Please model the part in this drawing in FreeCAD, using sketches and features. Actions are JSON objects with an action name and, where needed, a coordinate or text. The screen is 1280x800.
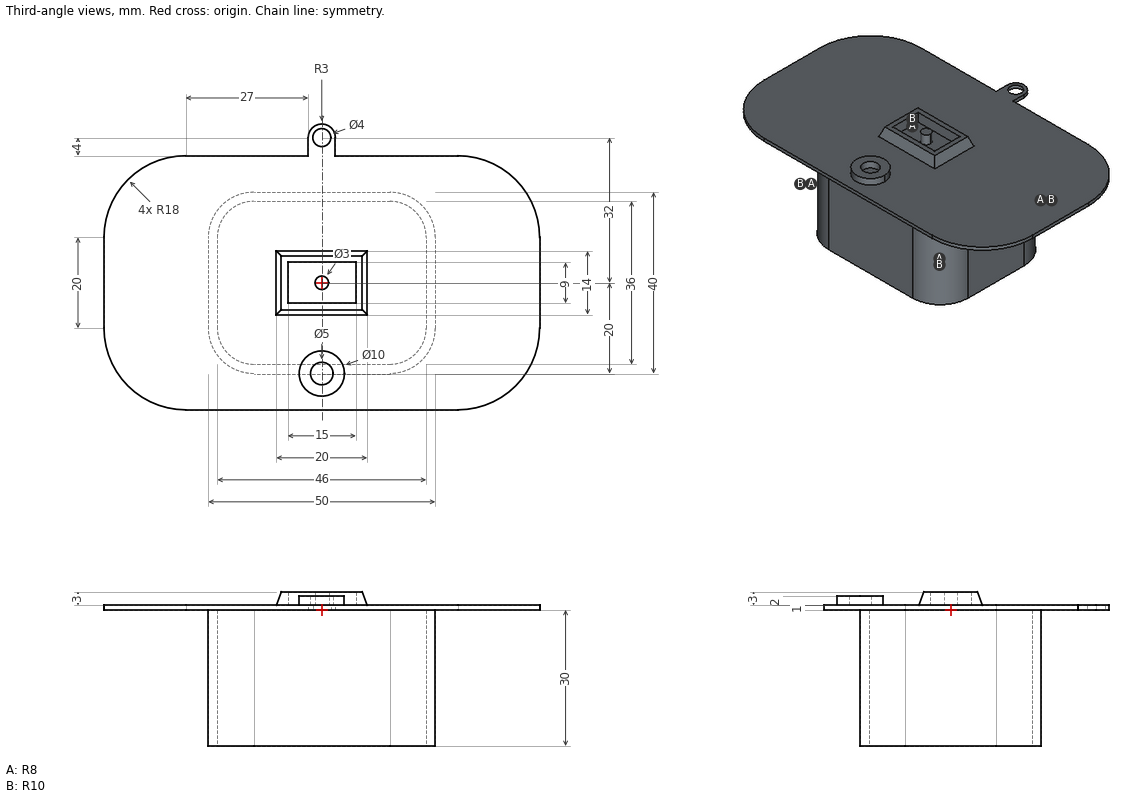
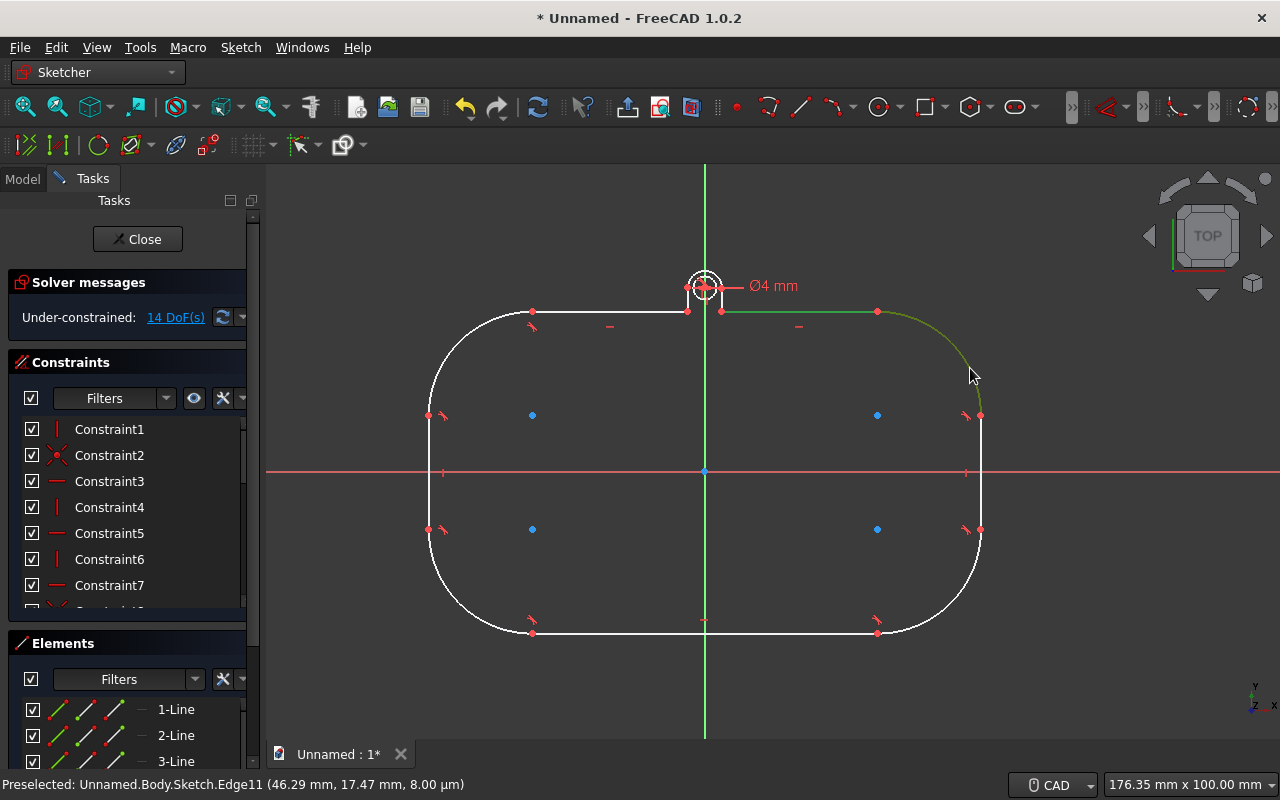
{"action": "key", "text": "t"}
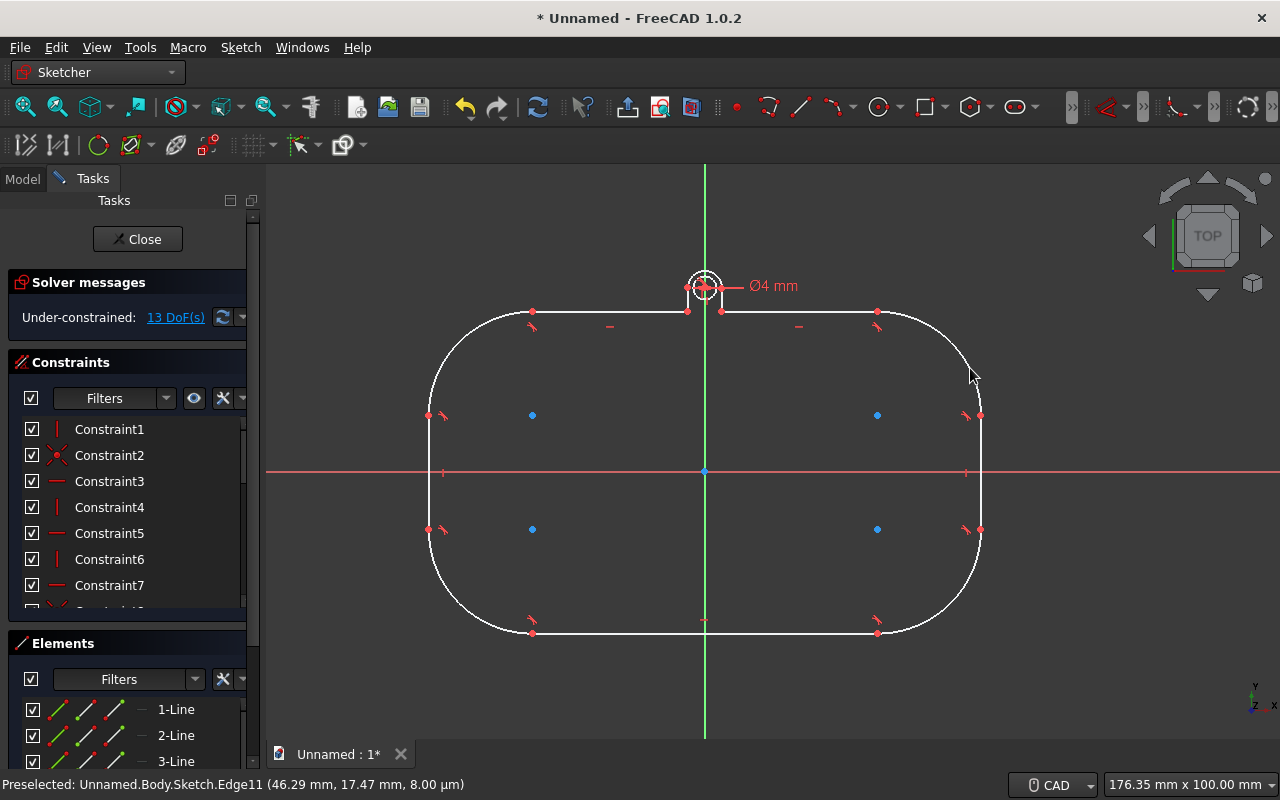
{"action": "scroll", "coordinate": [722, 303], "scroll_direction": "up", "scroll_amount": 3}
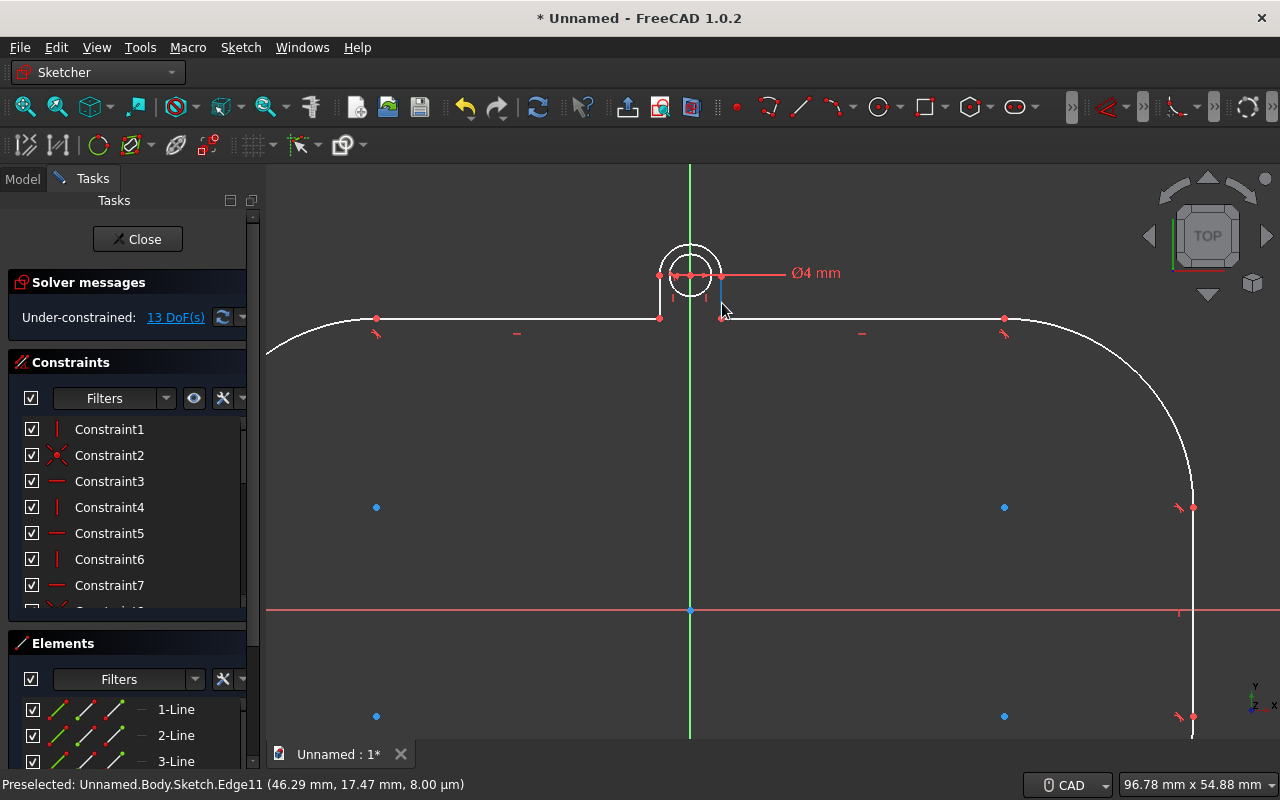
{"action": "left_click", "coordinate": [721, 302]}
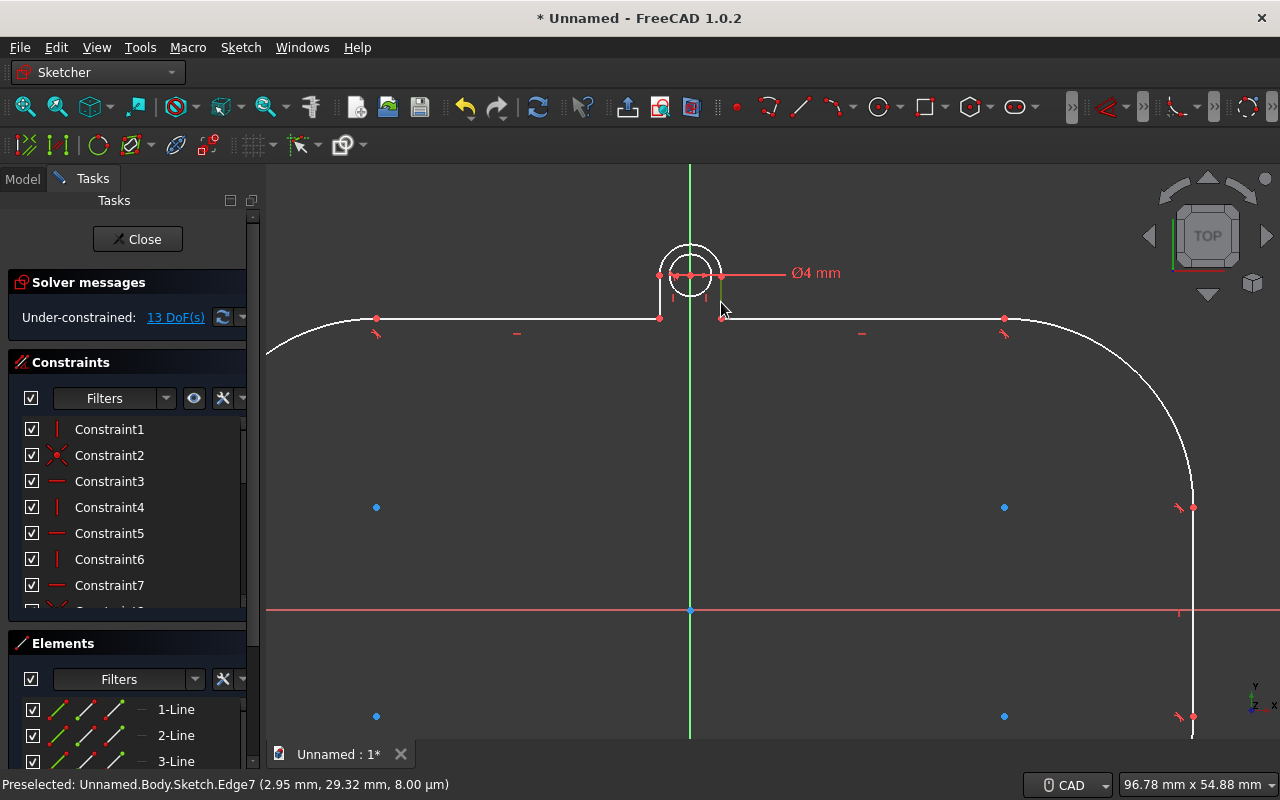
{"action": "scroll", "coordinate": [710, 251], "scroll_direction": "up", "scroll_amount": 2}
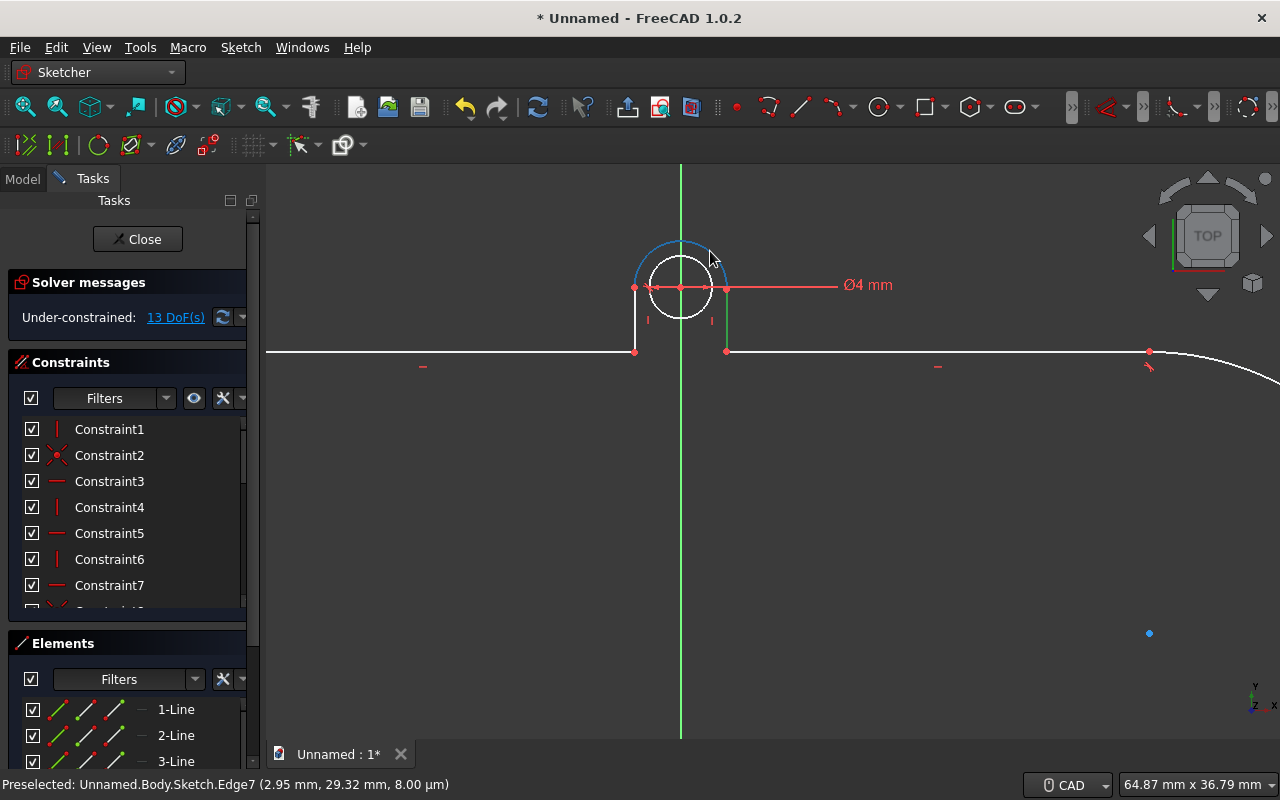
{"action": "left_click", "coordinate": [709, 251]}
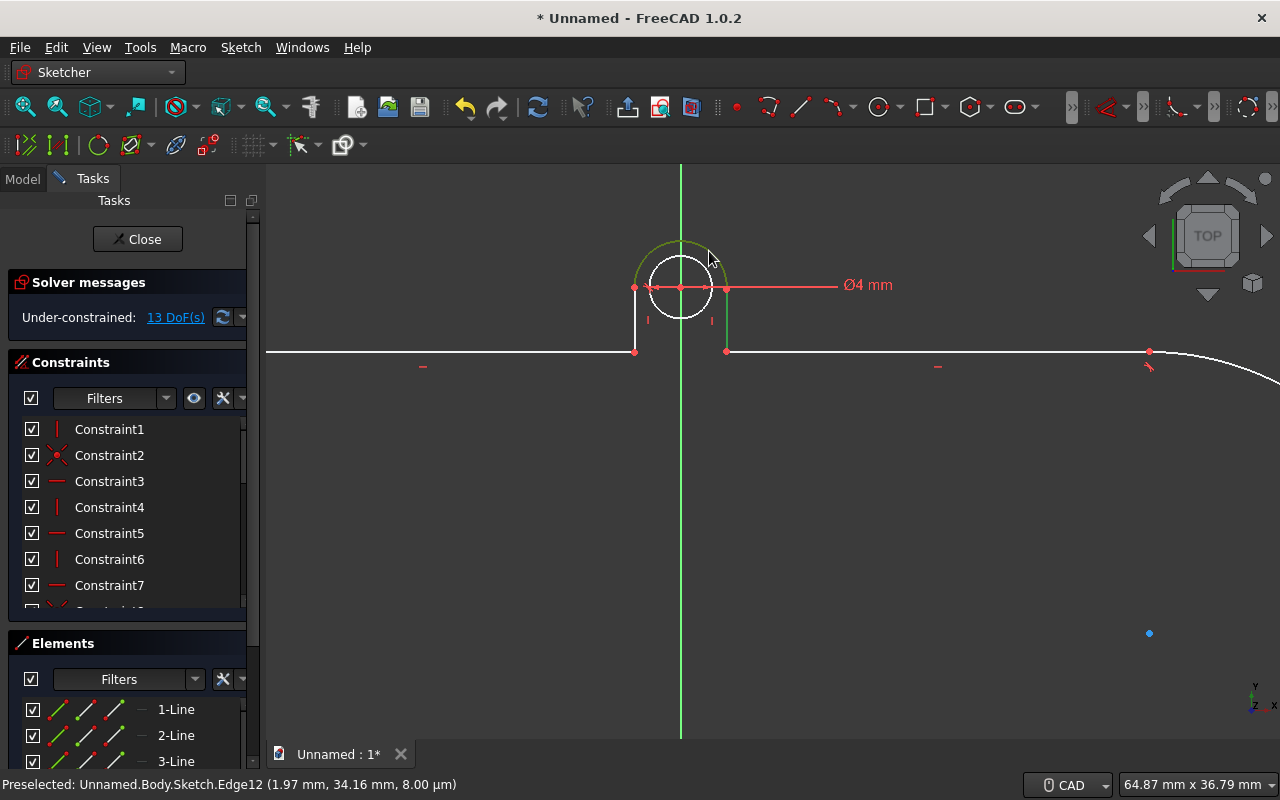
{"action": "key", "text": "t"}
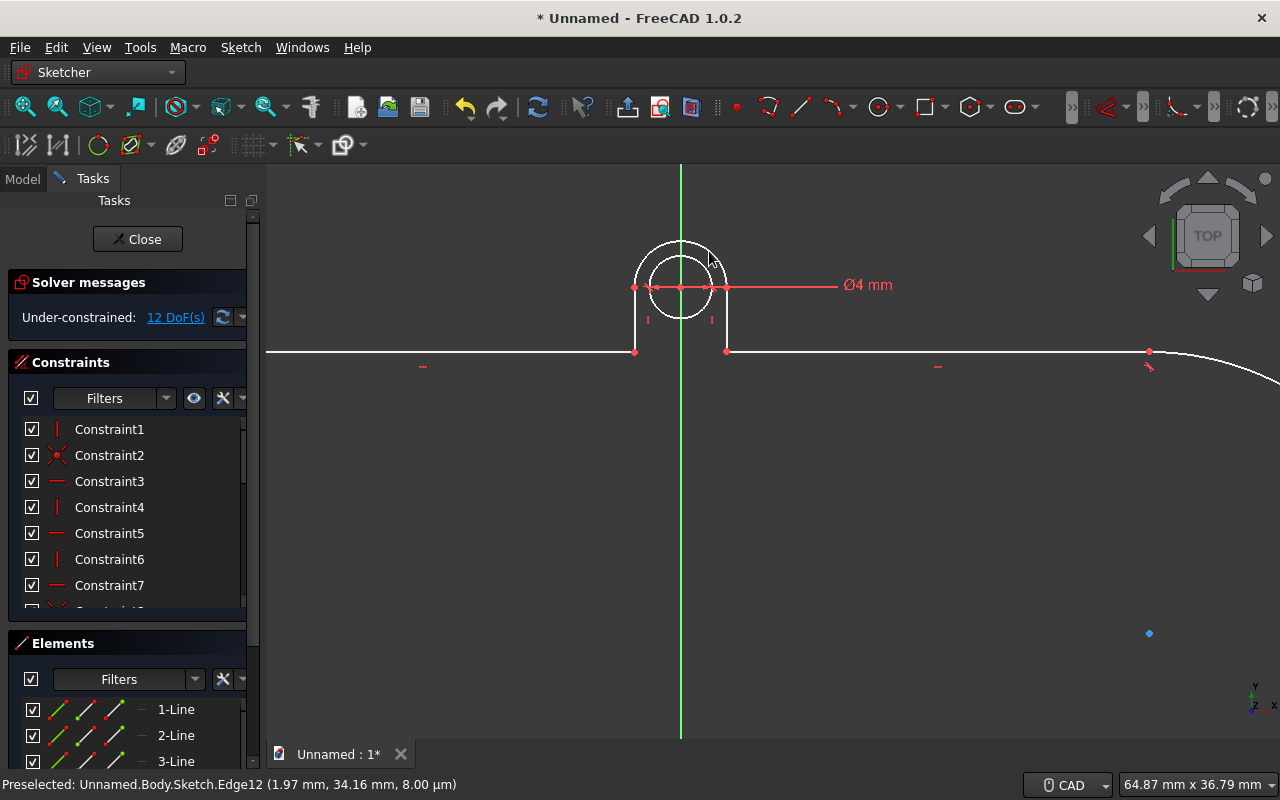
{"action": "scroll", "coordinate": [718, 288], "scroll_direction": "down", "scroll_amount": 5}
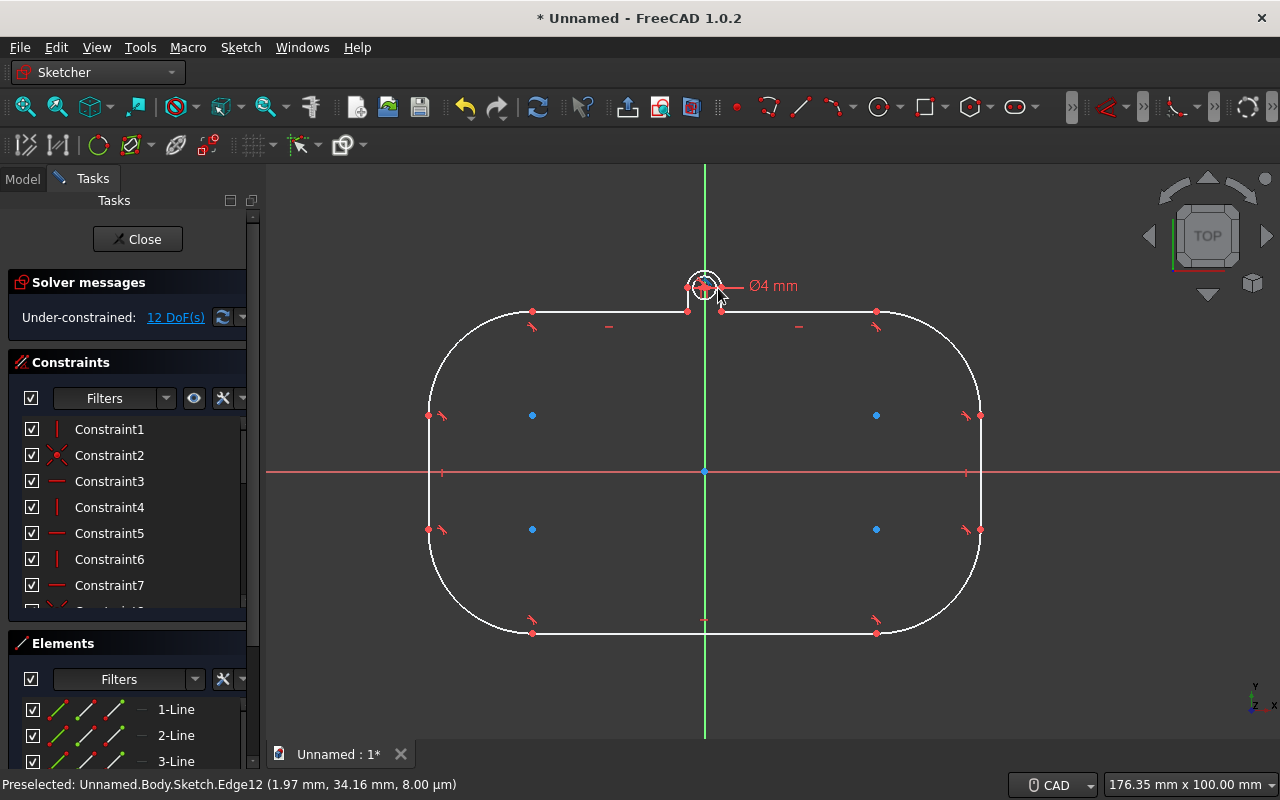
{"action": "left_click", "coordinate": [485, 323]}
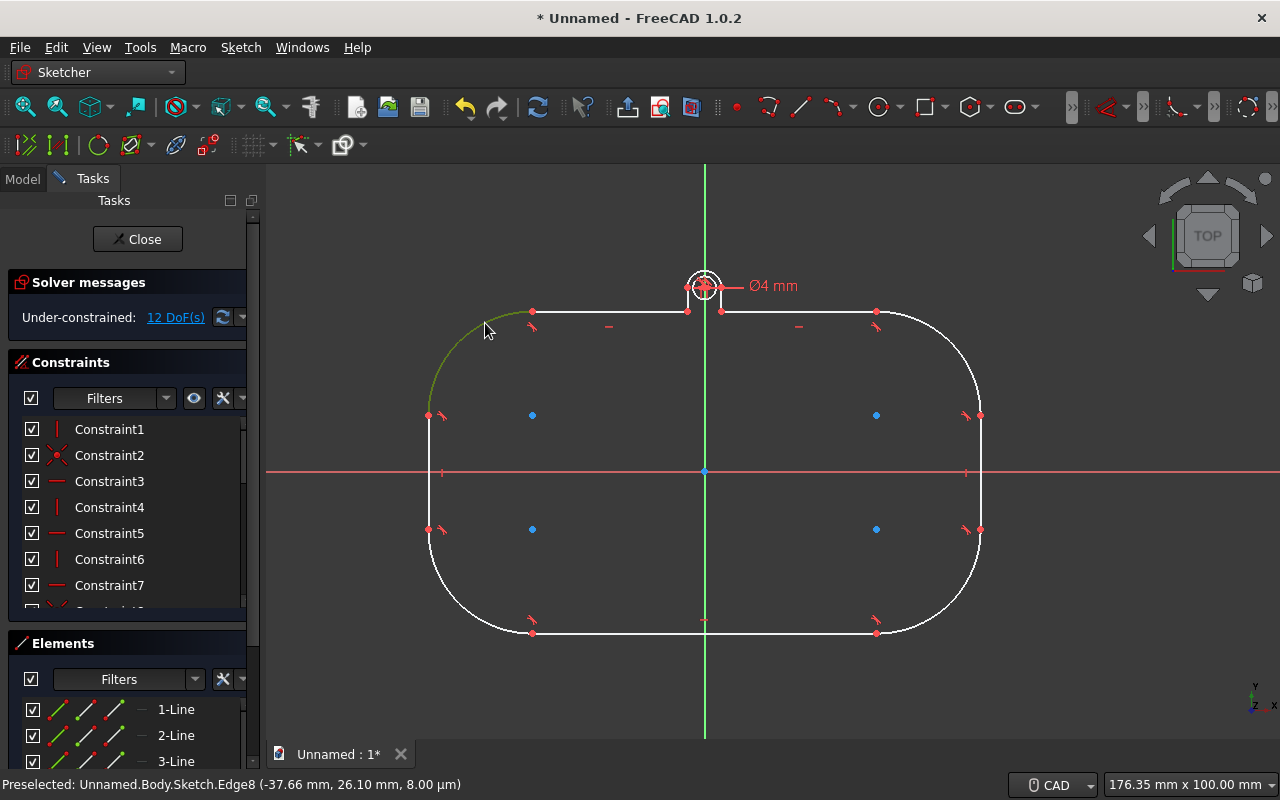
{"action": "left_click", "coordinate": [440, 577]}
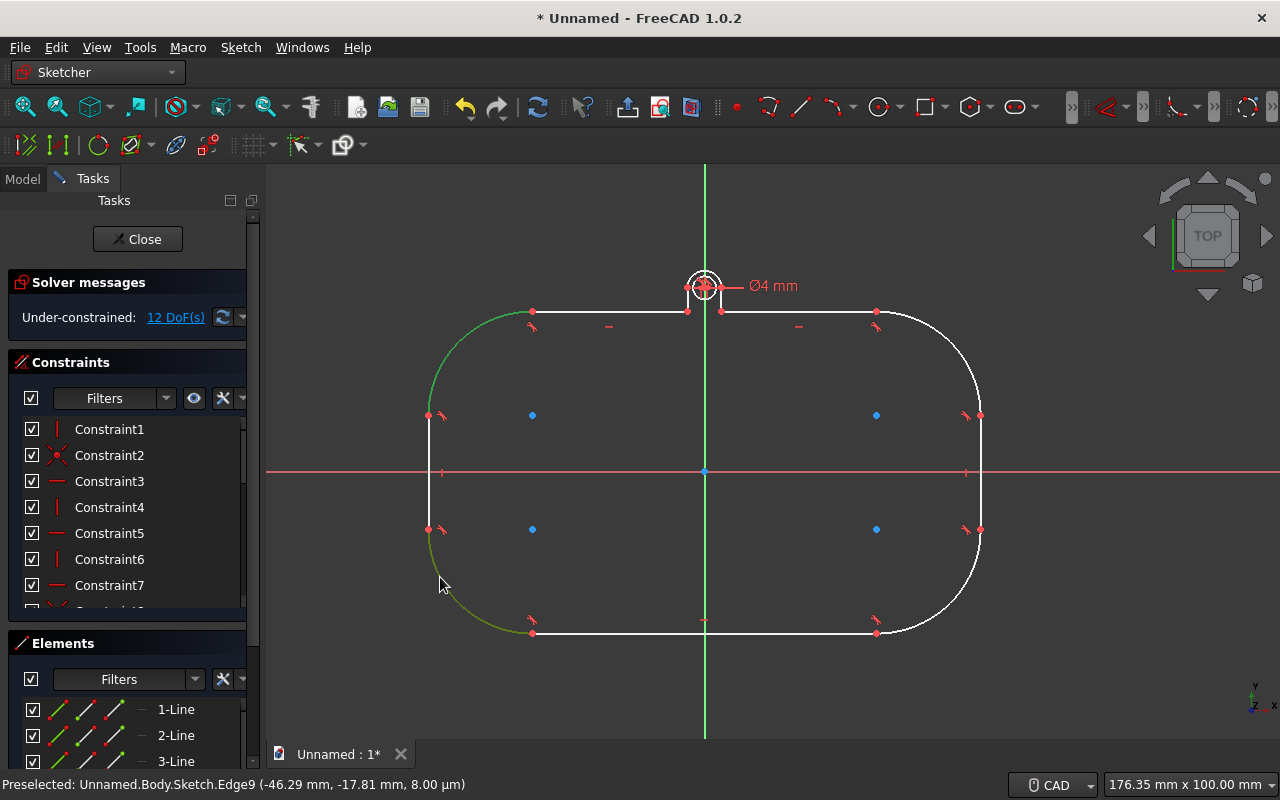
{"action": "left_click", "coordinate": [924, 622]}